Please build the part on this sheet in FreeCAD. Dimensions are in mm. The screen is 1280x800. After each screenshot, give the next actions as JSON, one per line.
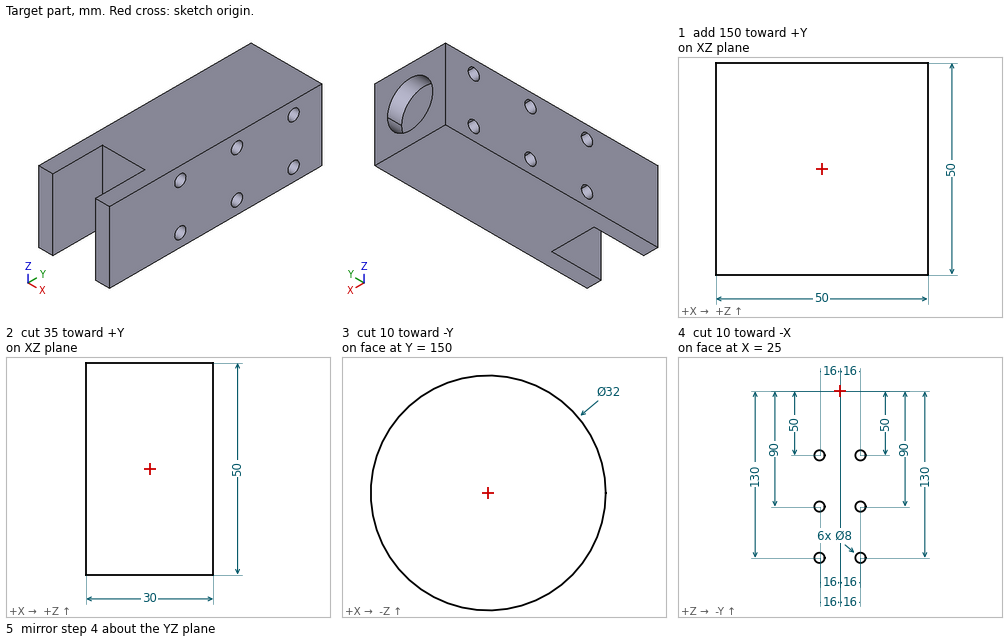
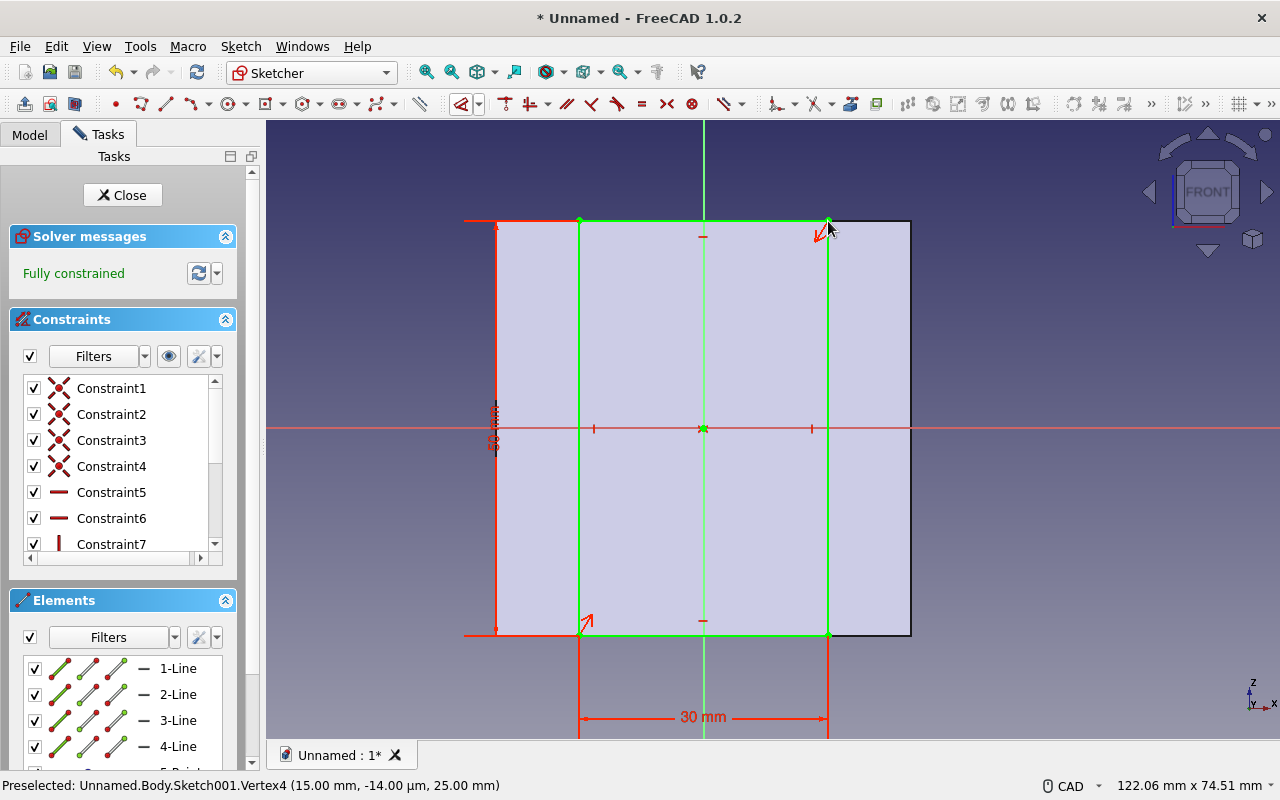
{"action": "left_click", "coordinate": [123, 195]}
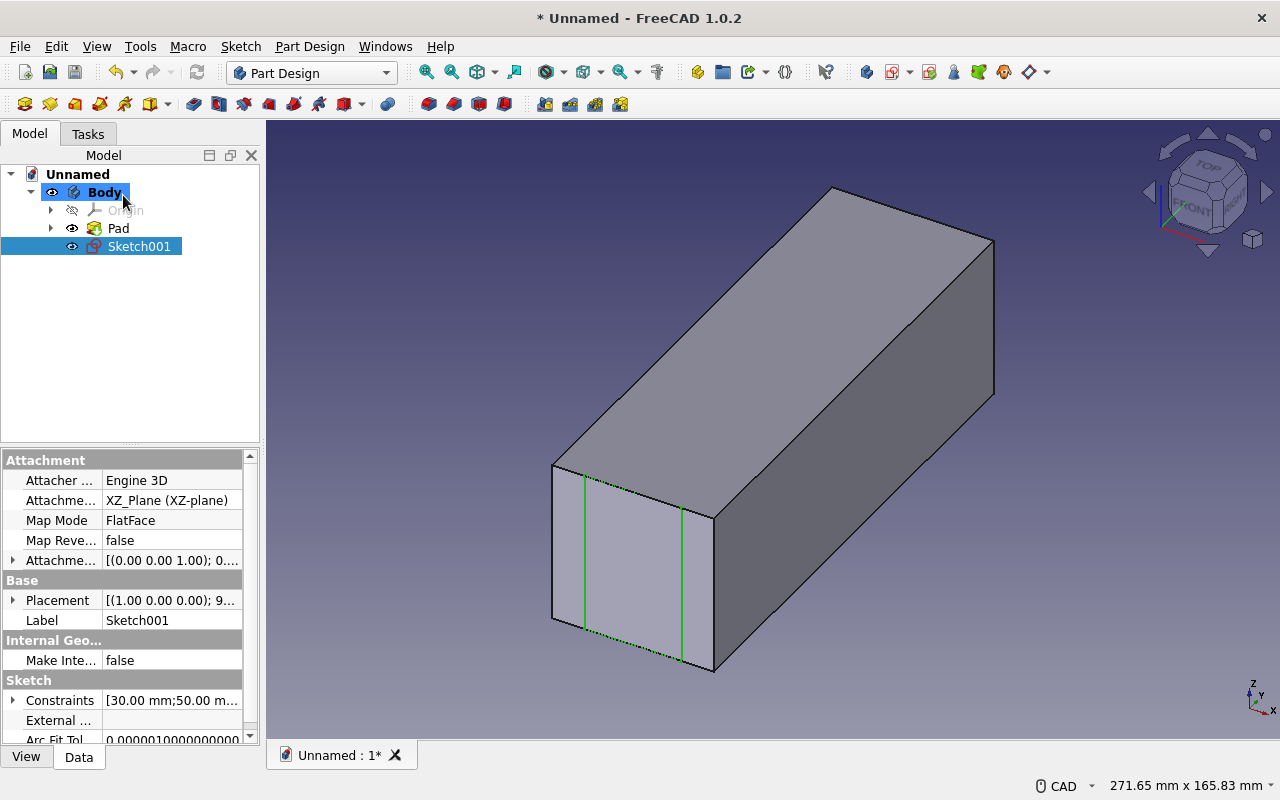
{"action": "left_click", "coordinate": [194, 104]}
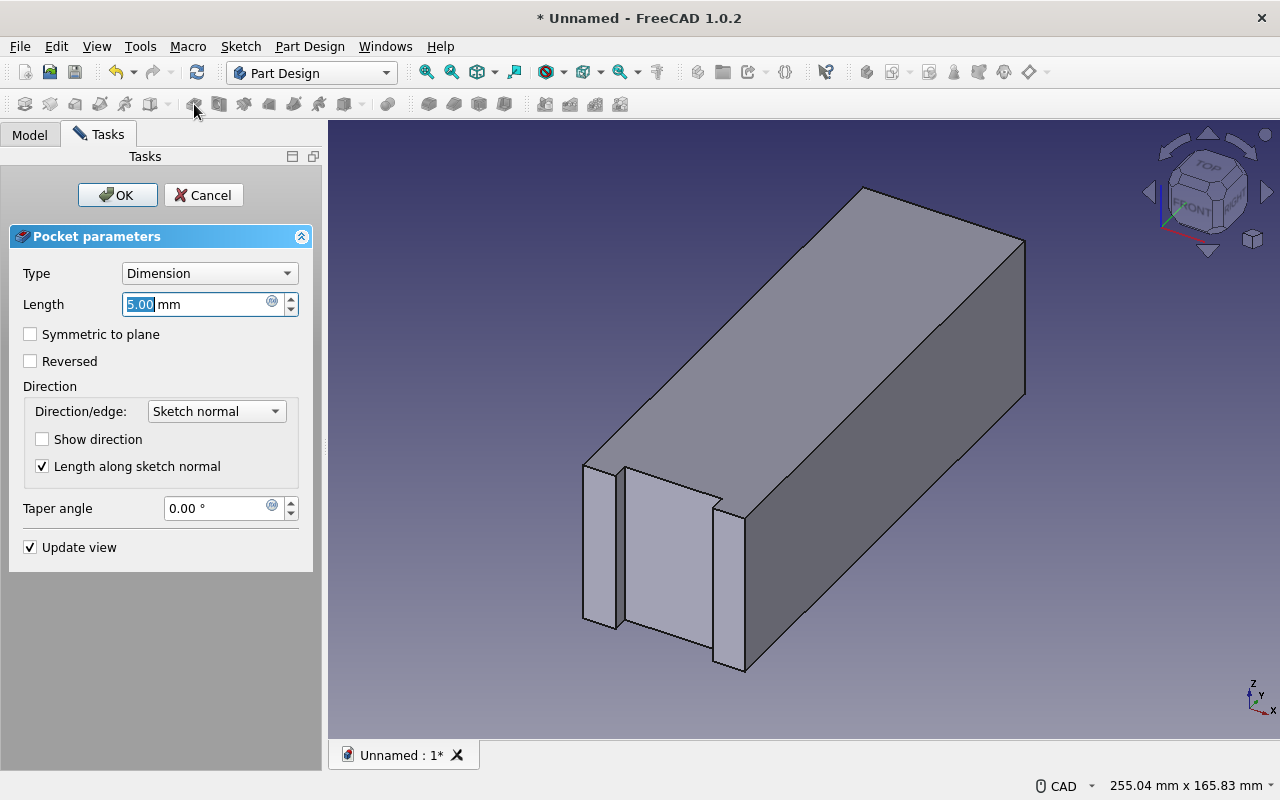
{"action": "type", "text": "35"}
{"action": "key", "text": "Tab"}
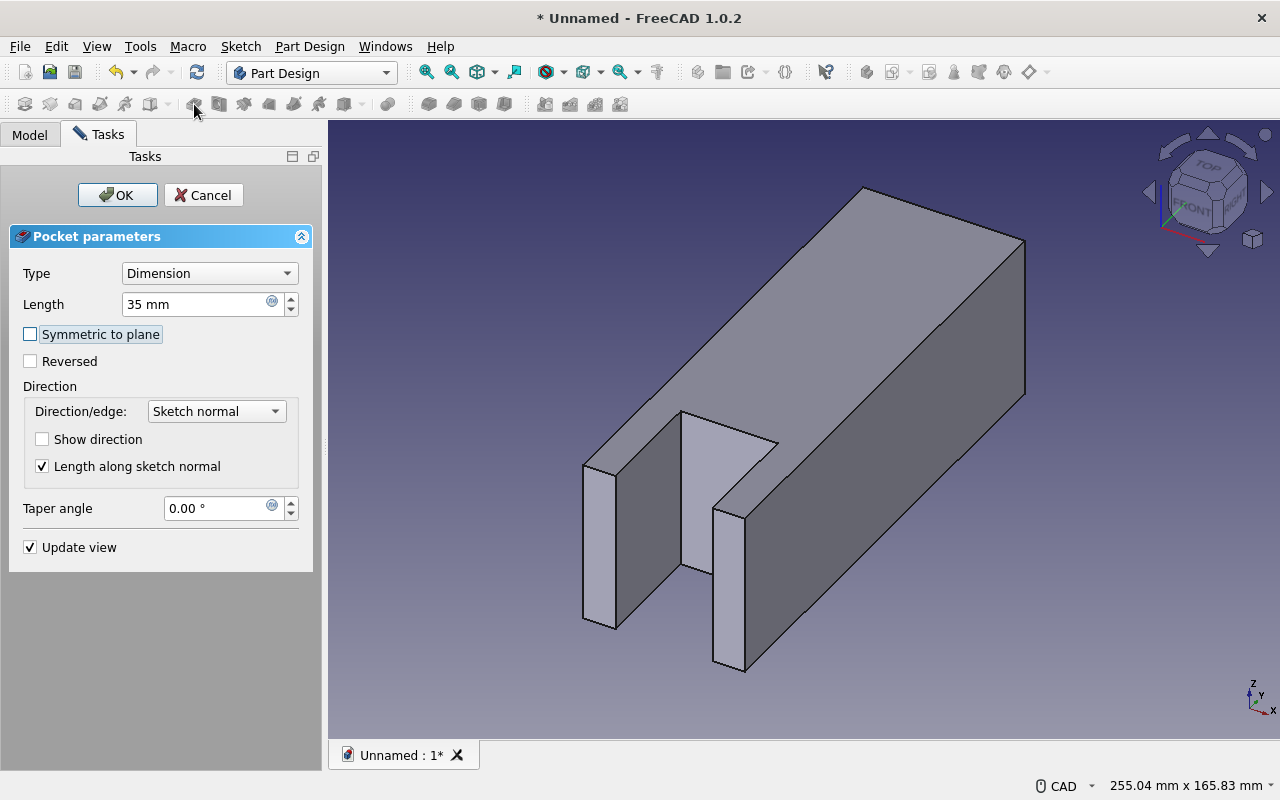
{"action": "left_click", "coordinate": [118, 195]}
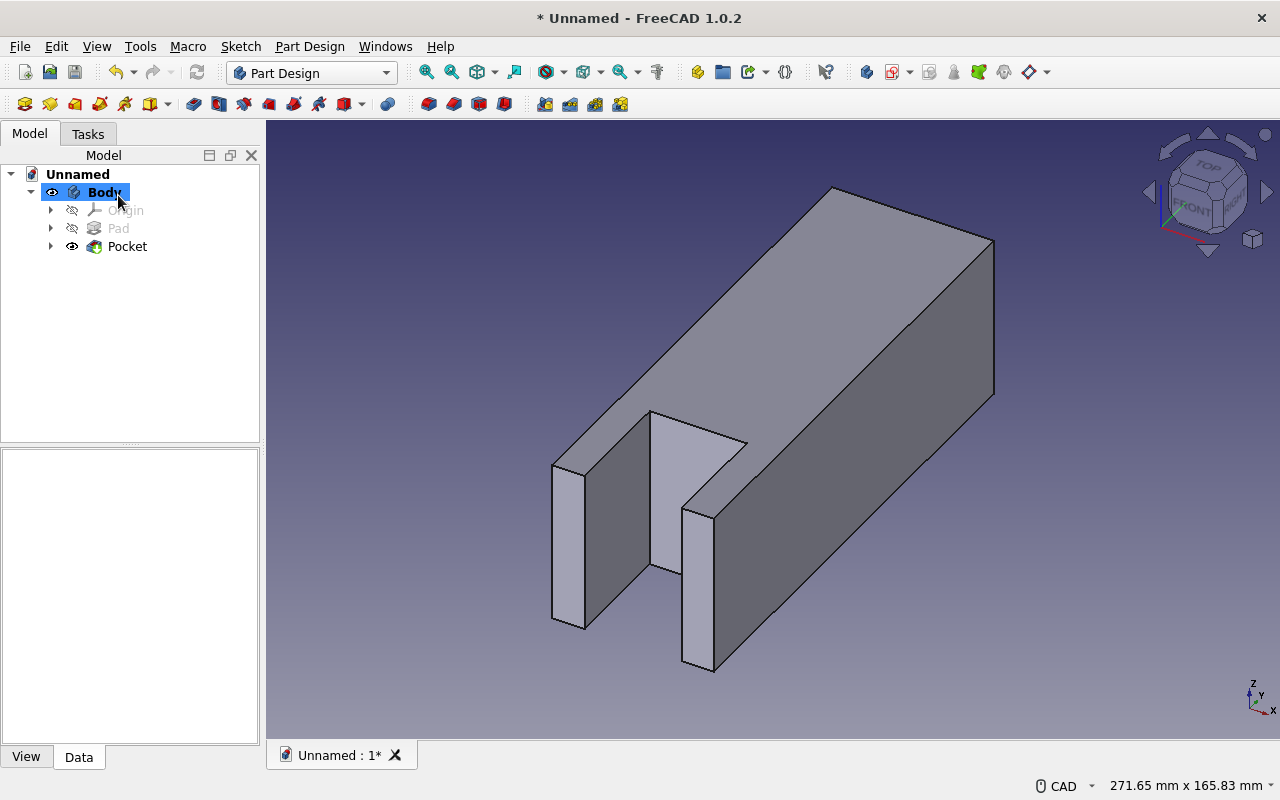
{"action": "key", "text": "4"}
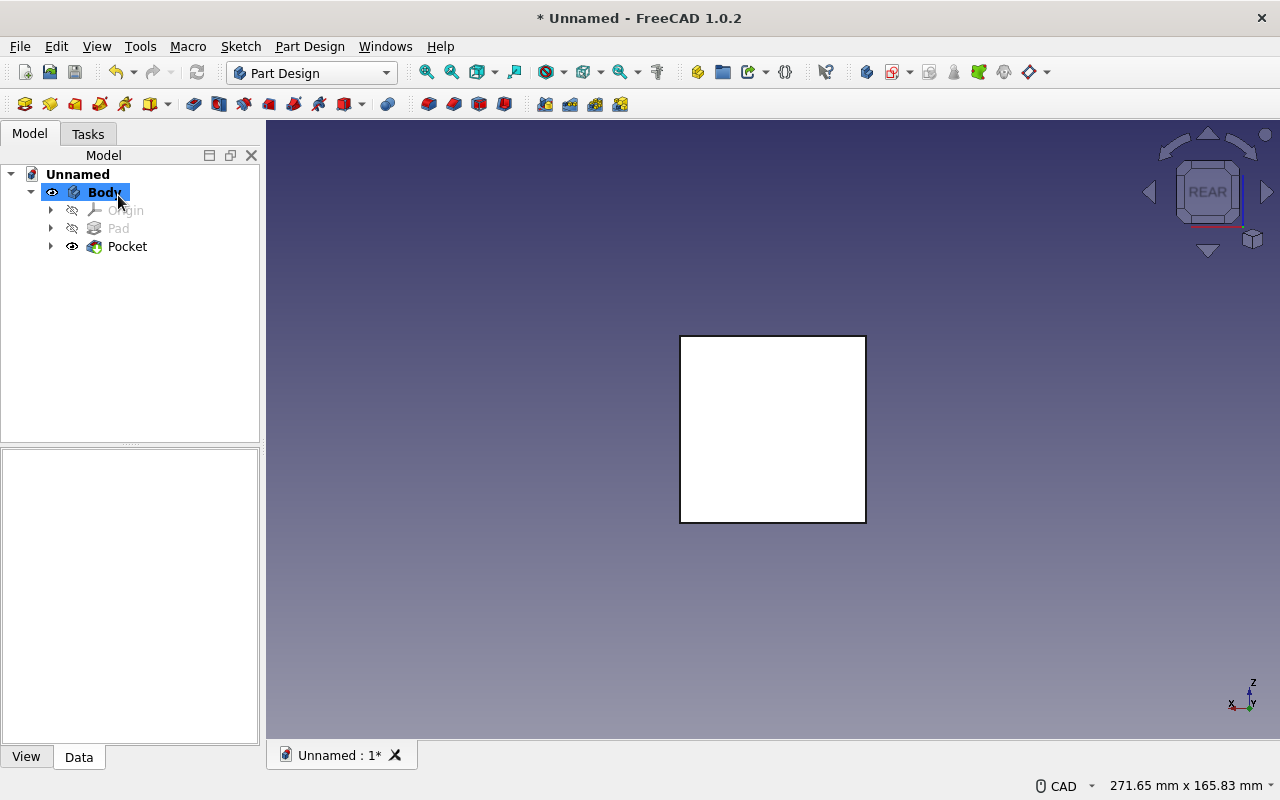
{"action": "left_click", "coordinate": [427, 72]}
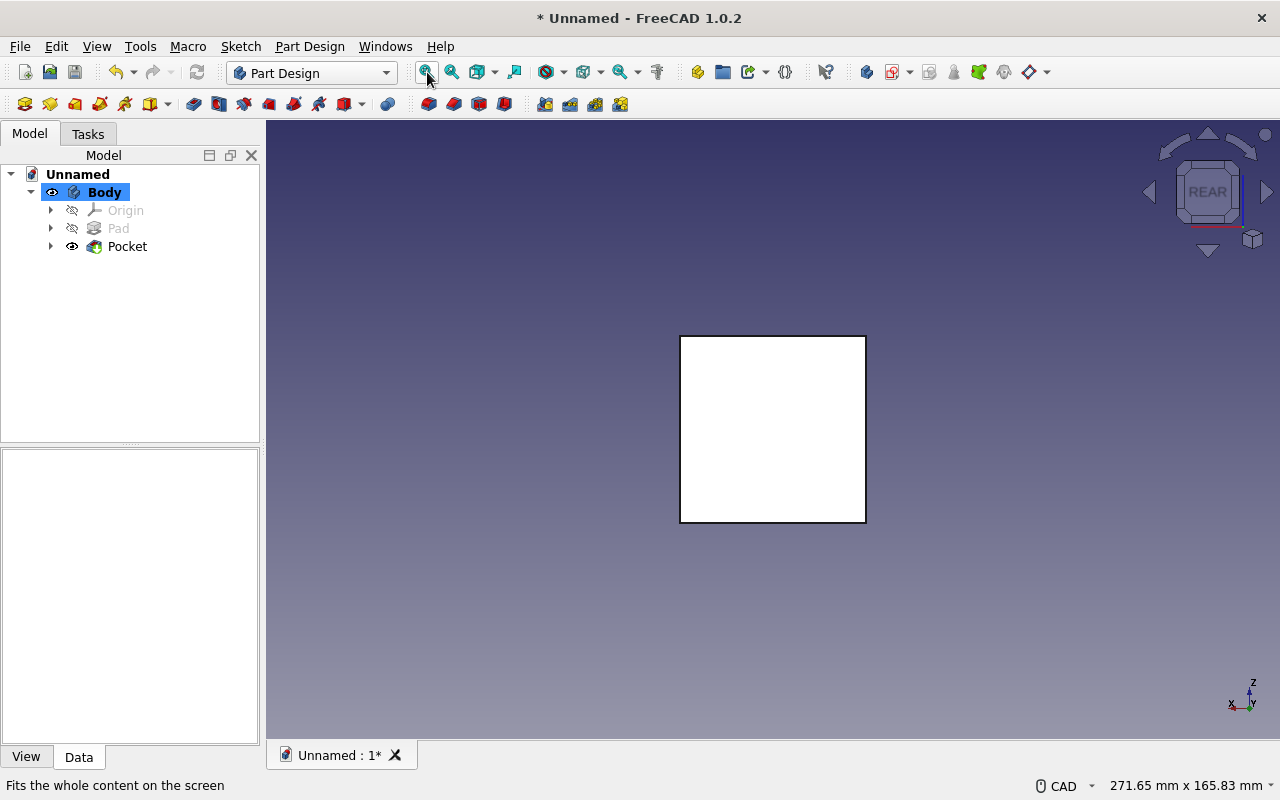
{"action": "left_click", "coordinate": [773, 429]}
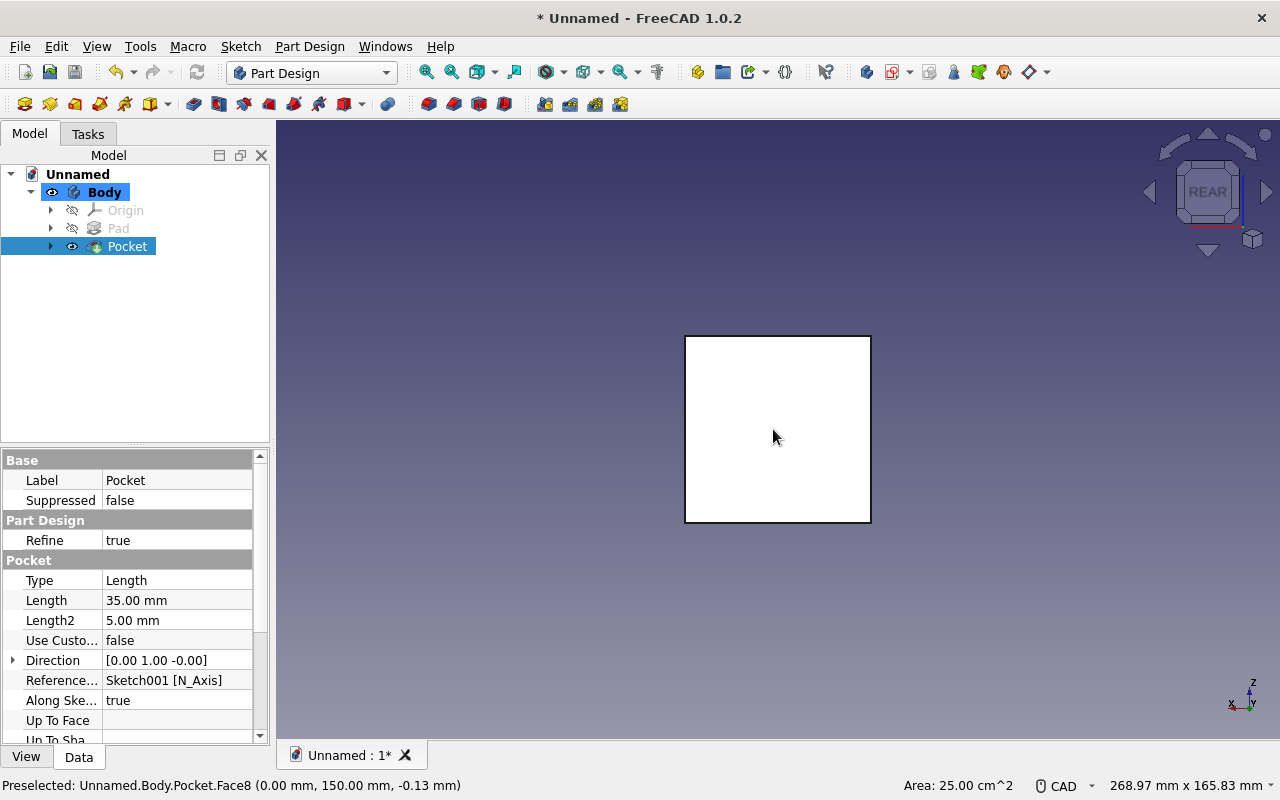
{"action": "left_click", "coordinate": [892, 72]}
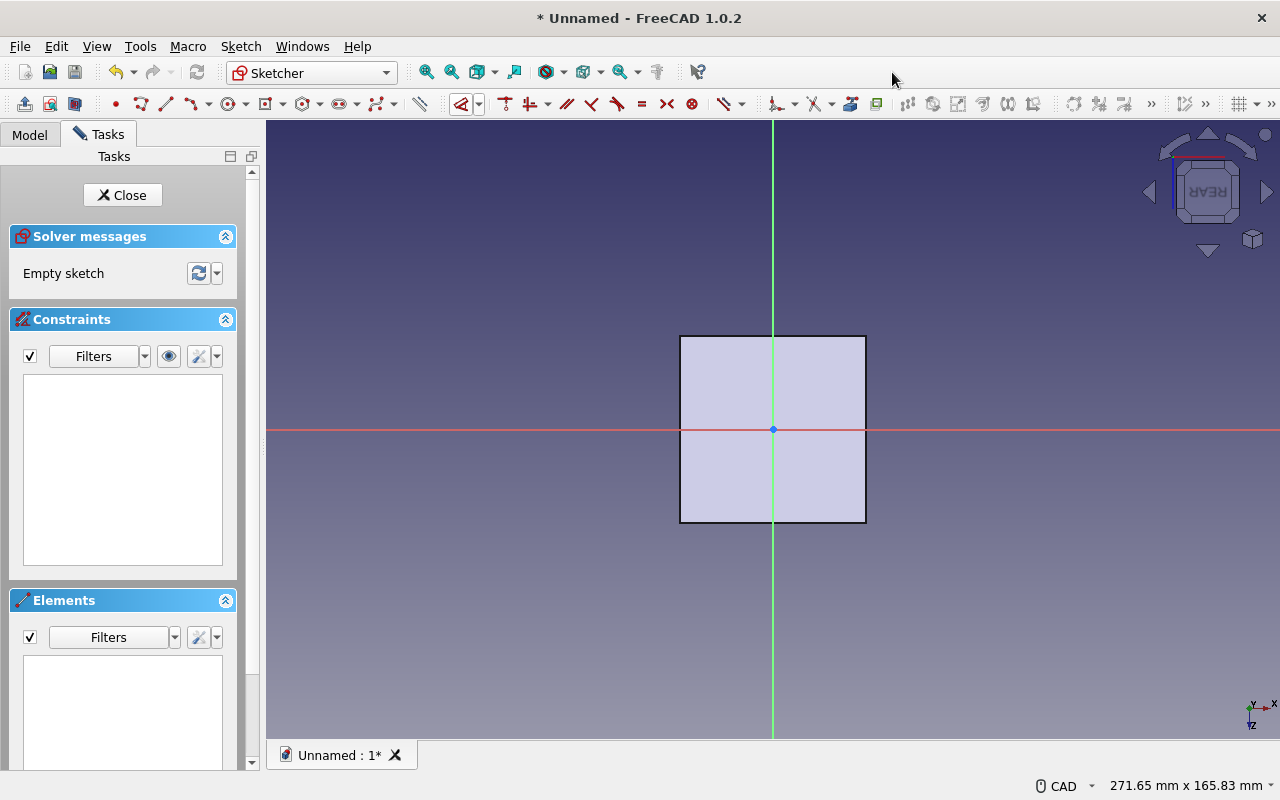
{"action": "scroll", "coordinate": [803, 429], "scroll_direction": "up", "scroll_amount": 6}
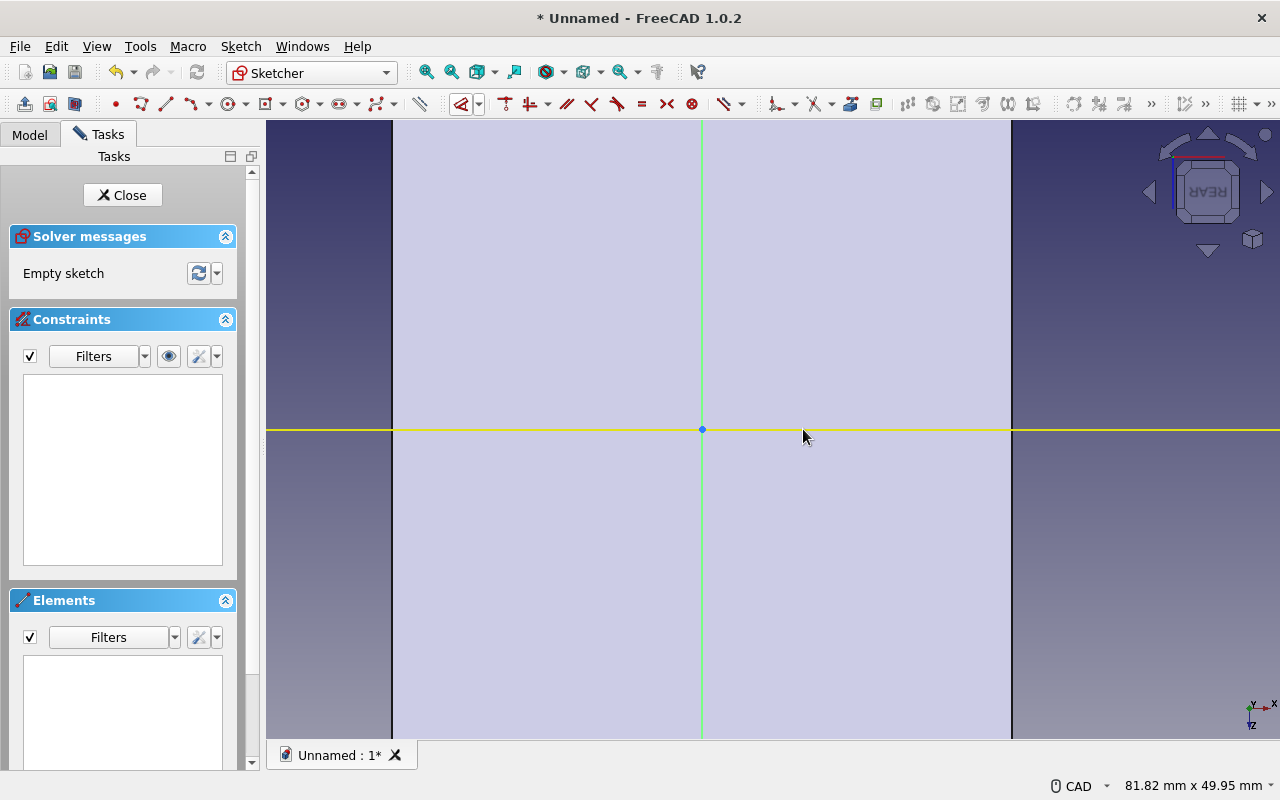
{"action": "left_click", "coordinate": [228, 104]}